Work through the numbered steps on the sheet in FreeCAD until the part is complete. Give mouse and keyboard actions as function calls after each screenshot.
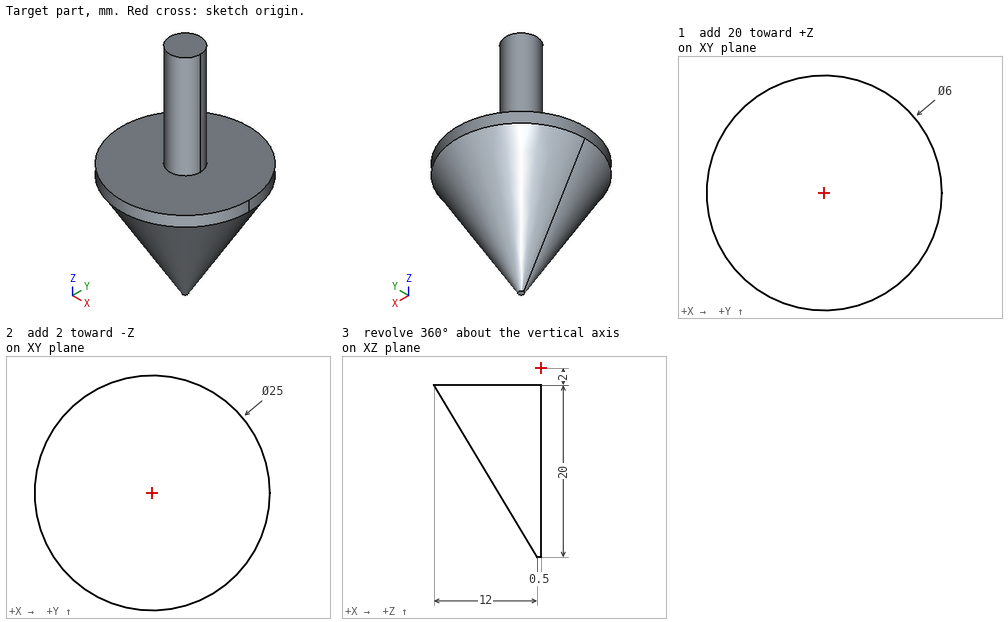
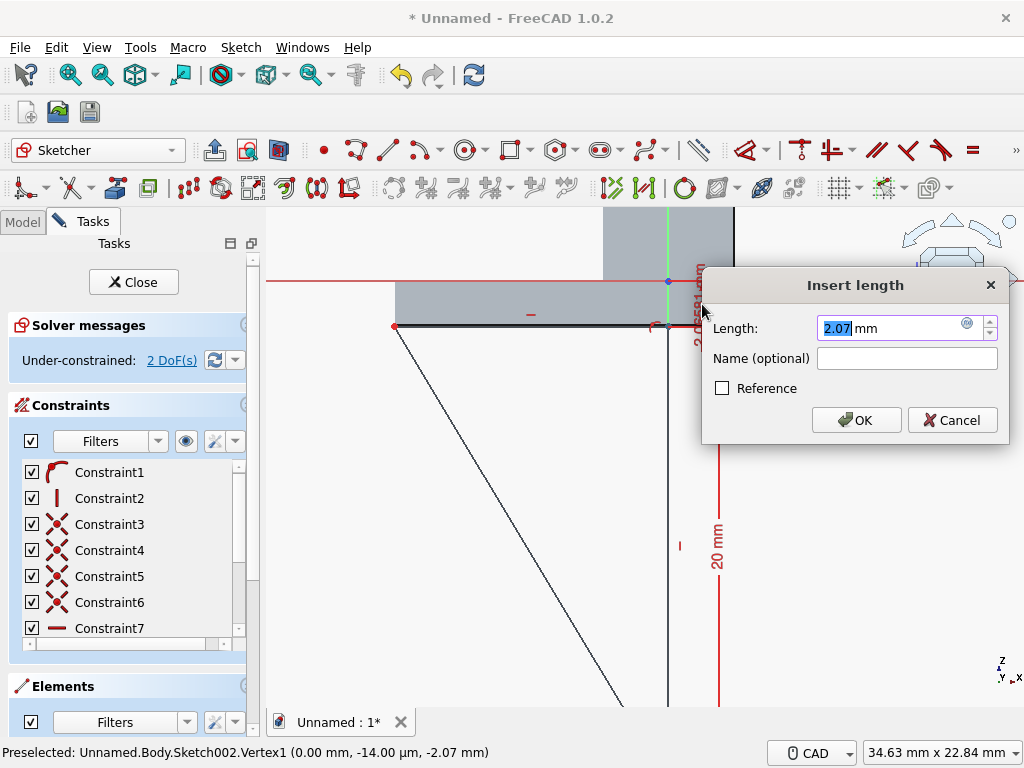
text(2)
key(Return)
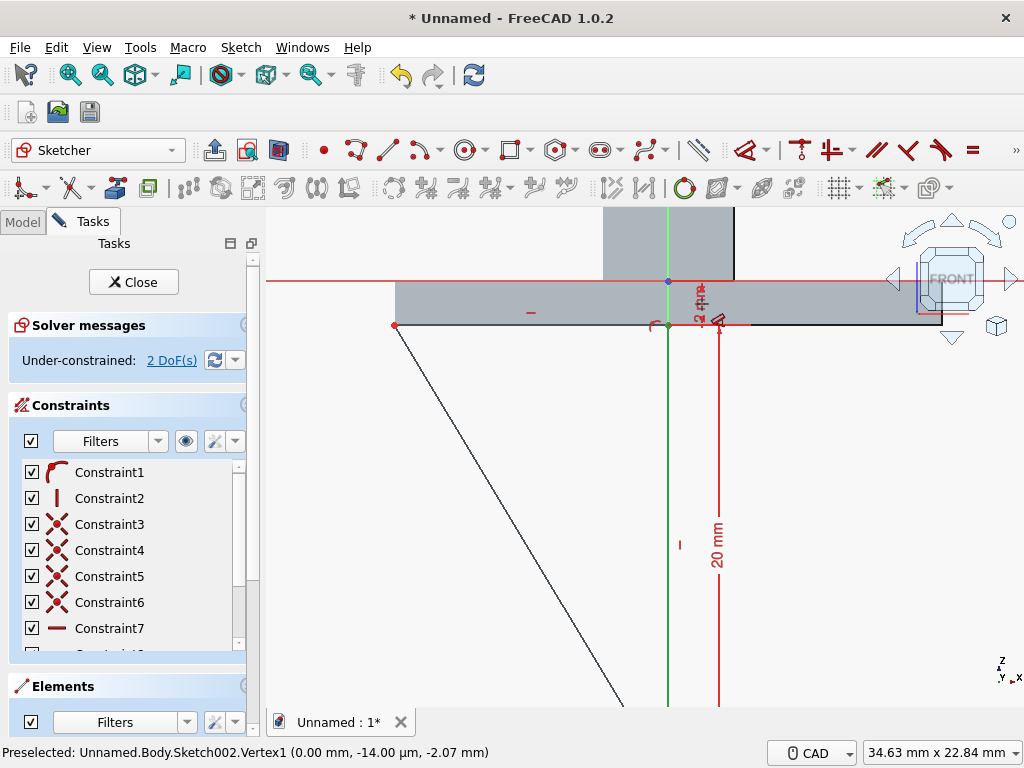
scroll(668, 324, down, 2)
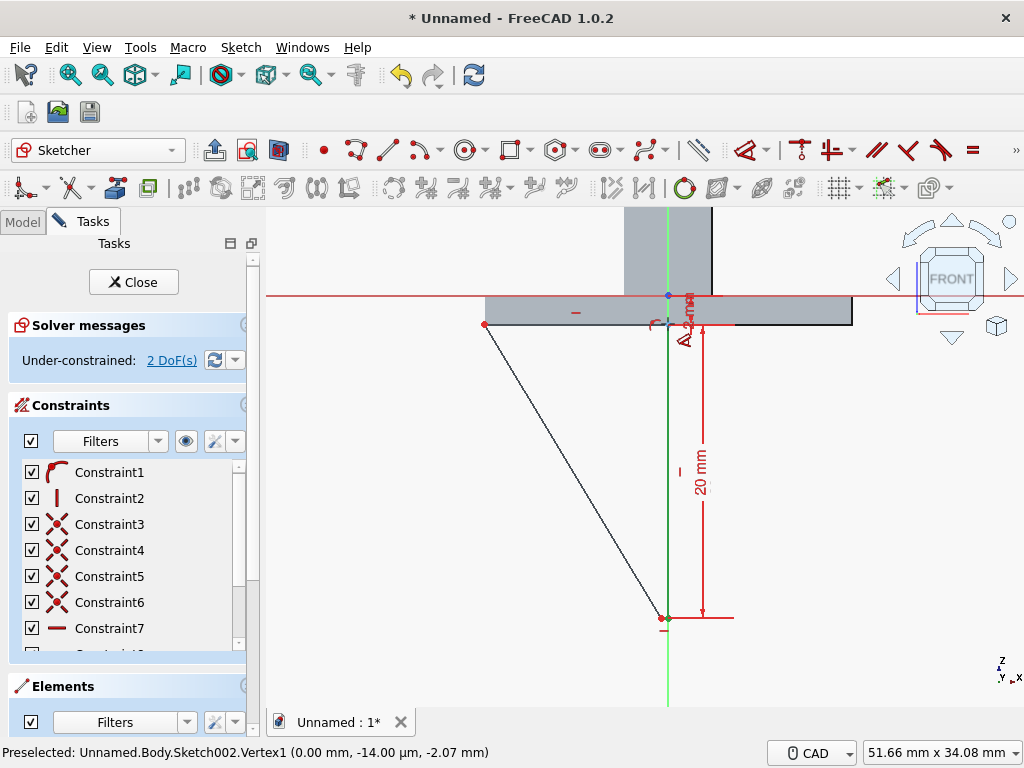
scroll(665, 618, up, 9)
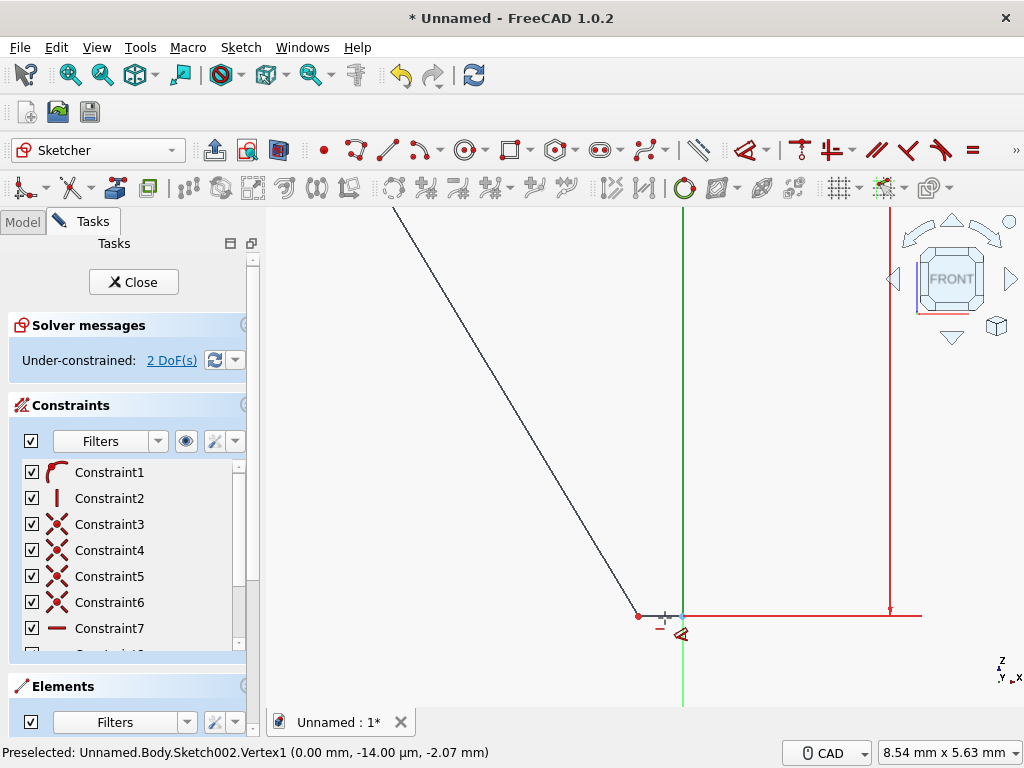
click(661, 616)
click(661, 650)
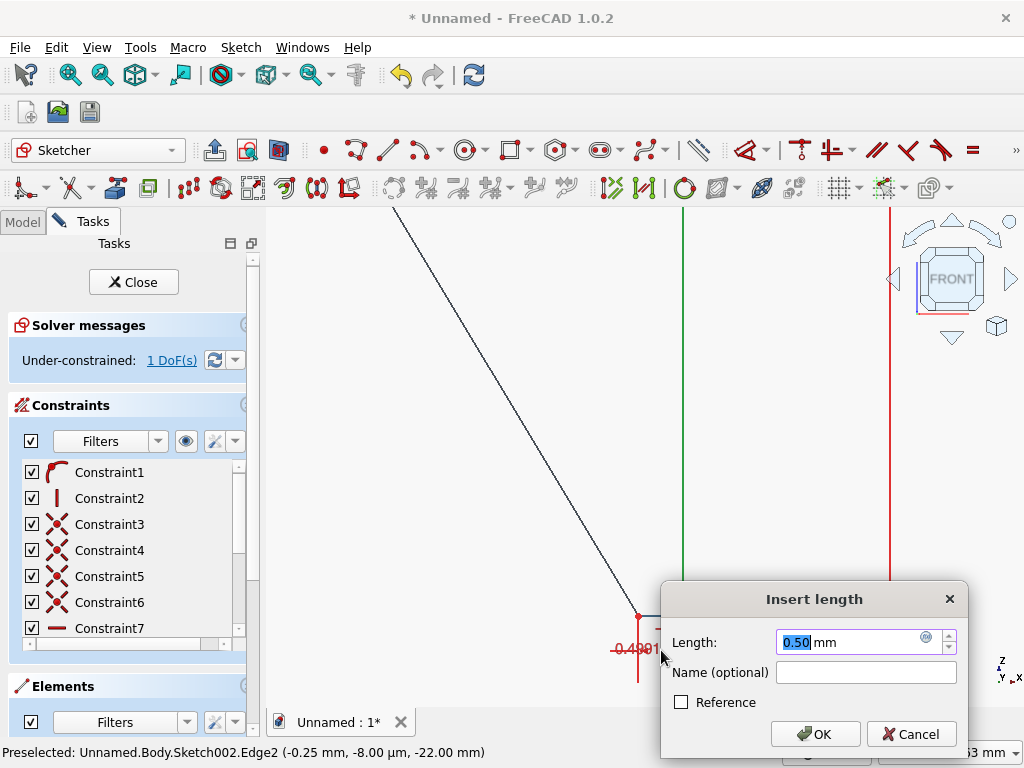
text(0.5)
key(Return)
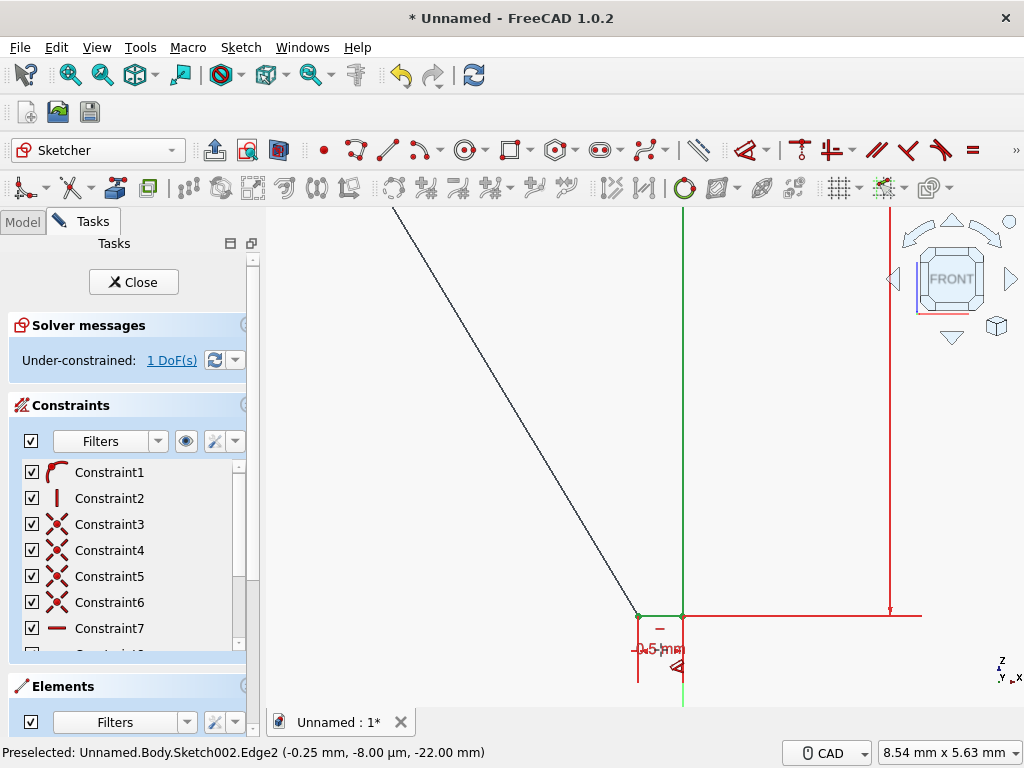
scroll(665, 619, down, 9)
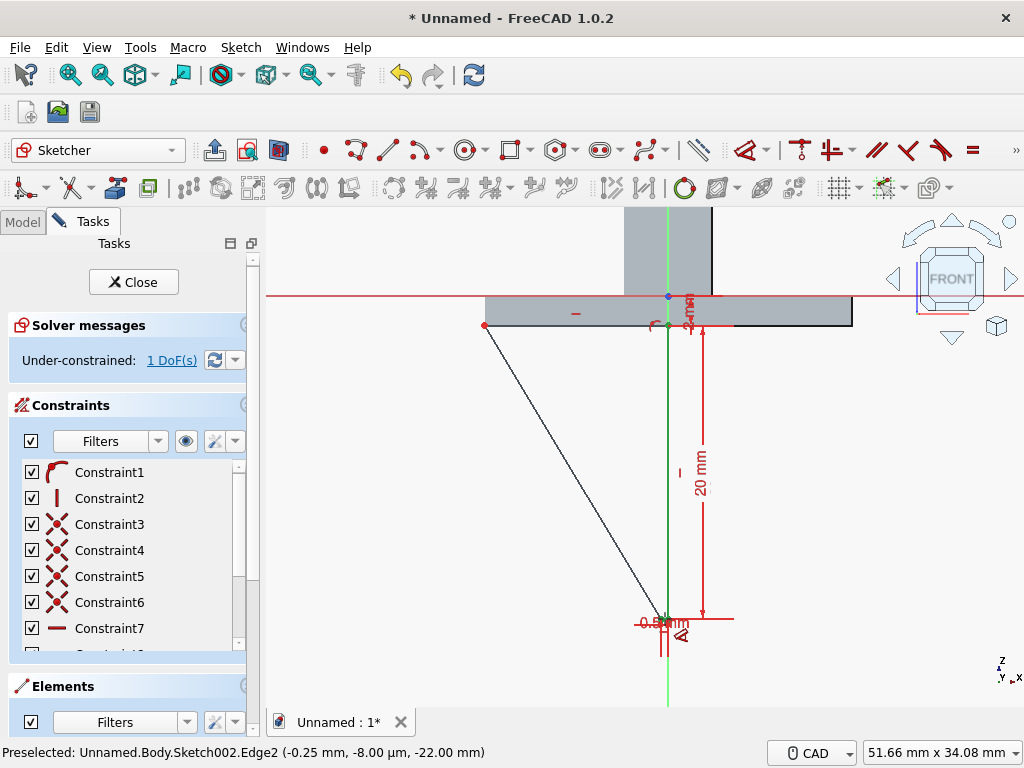
click(626, 561)
click(573, 653)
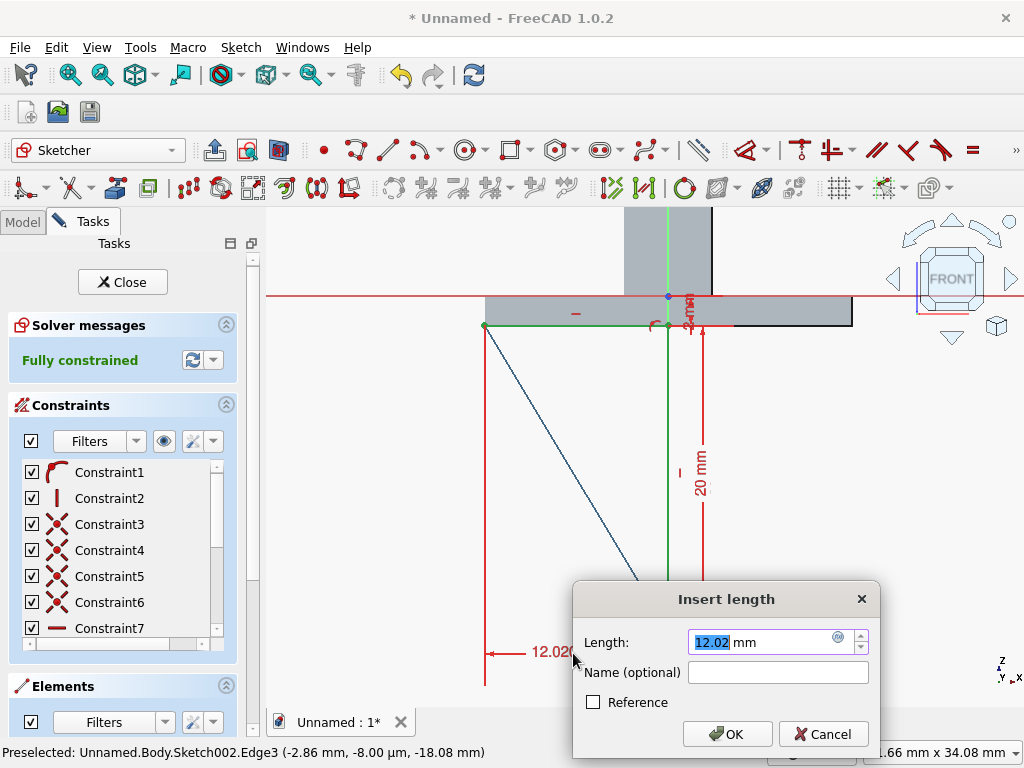
text(12)
key(Return)
key(Escape)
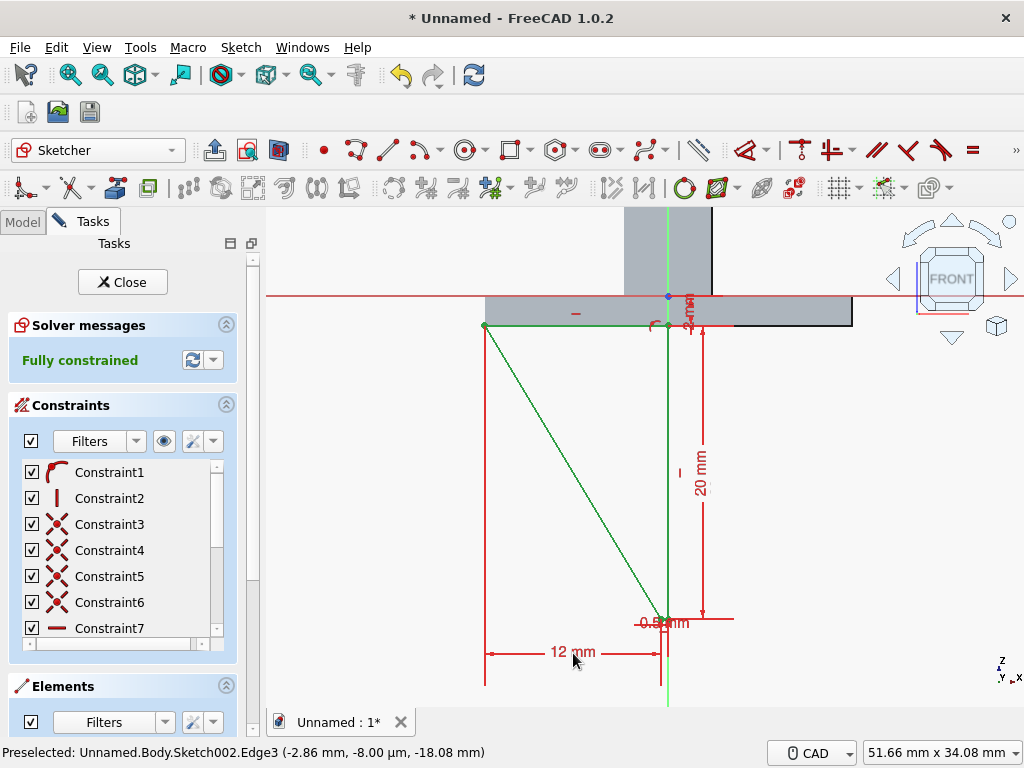
click(123, 282)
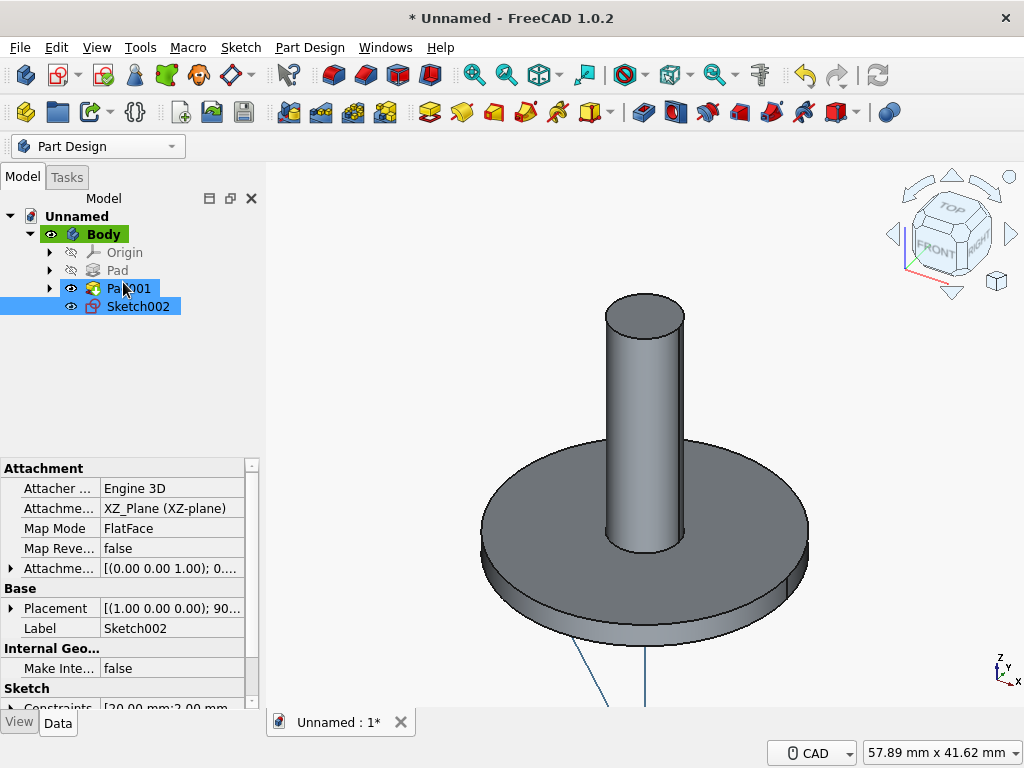
click(462, 112)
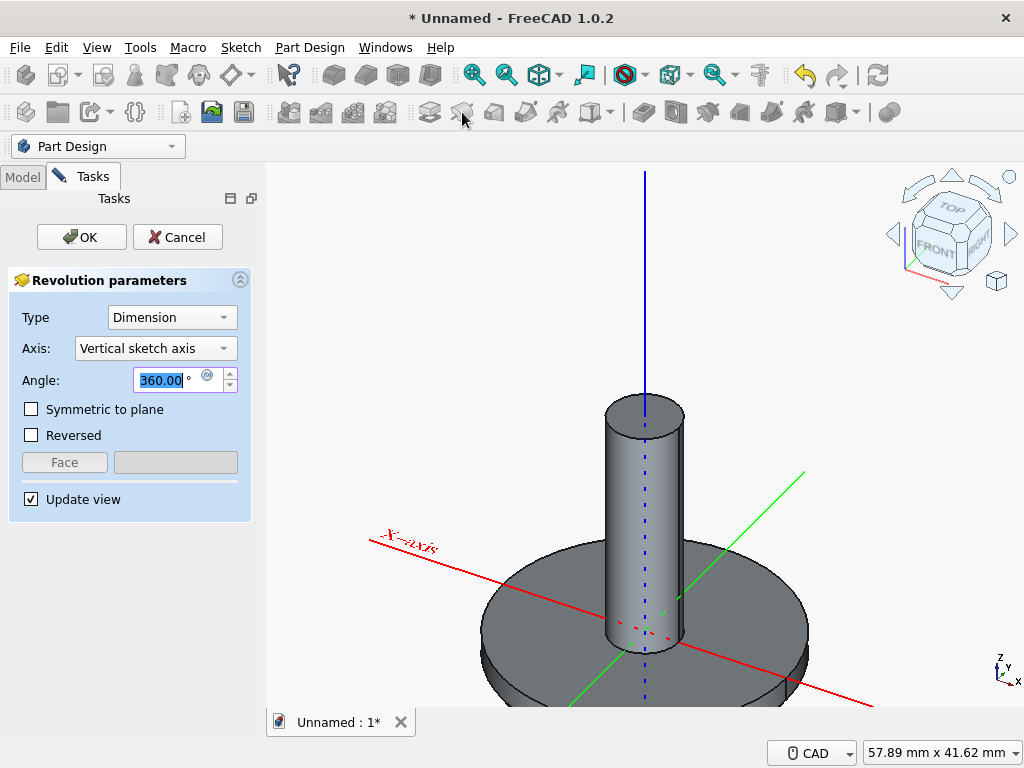
click(82, 237)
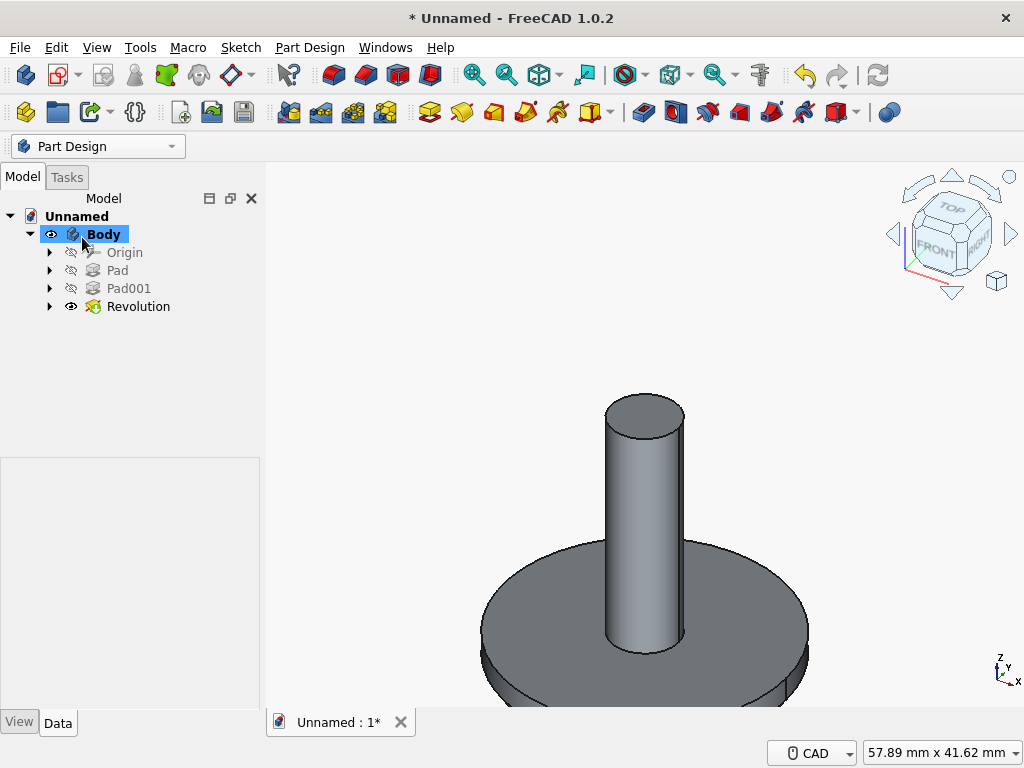
key(0)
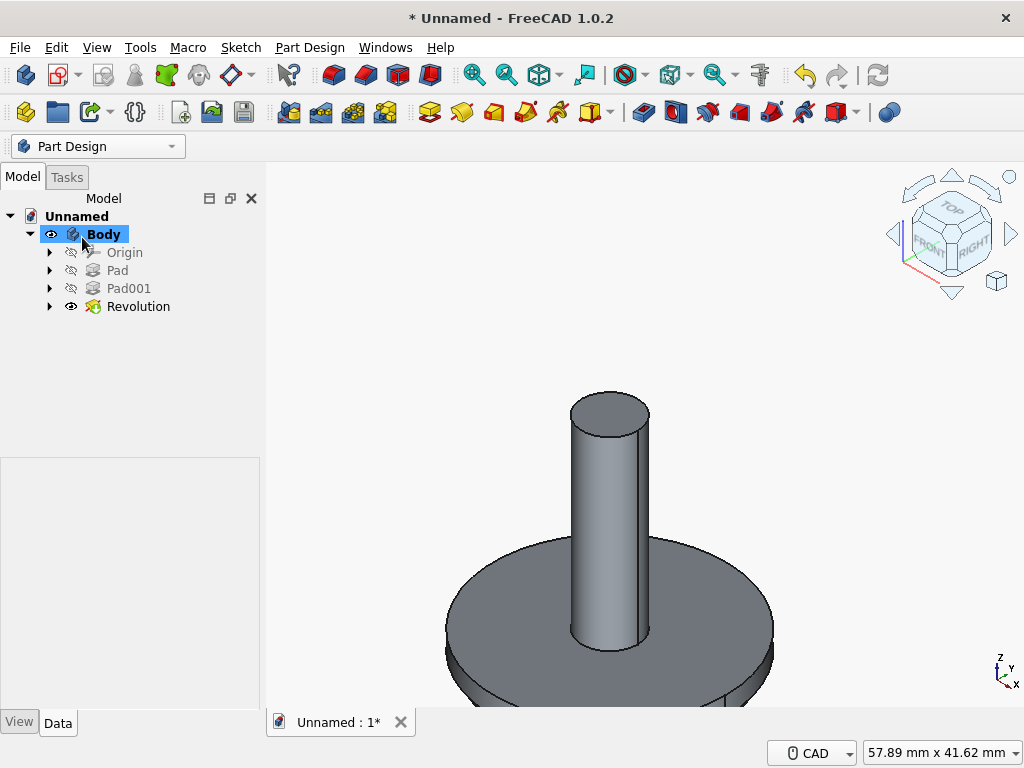
click(476, 76)